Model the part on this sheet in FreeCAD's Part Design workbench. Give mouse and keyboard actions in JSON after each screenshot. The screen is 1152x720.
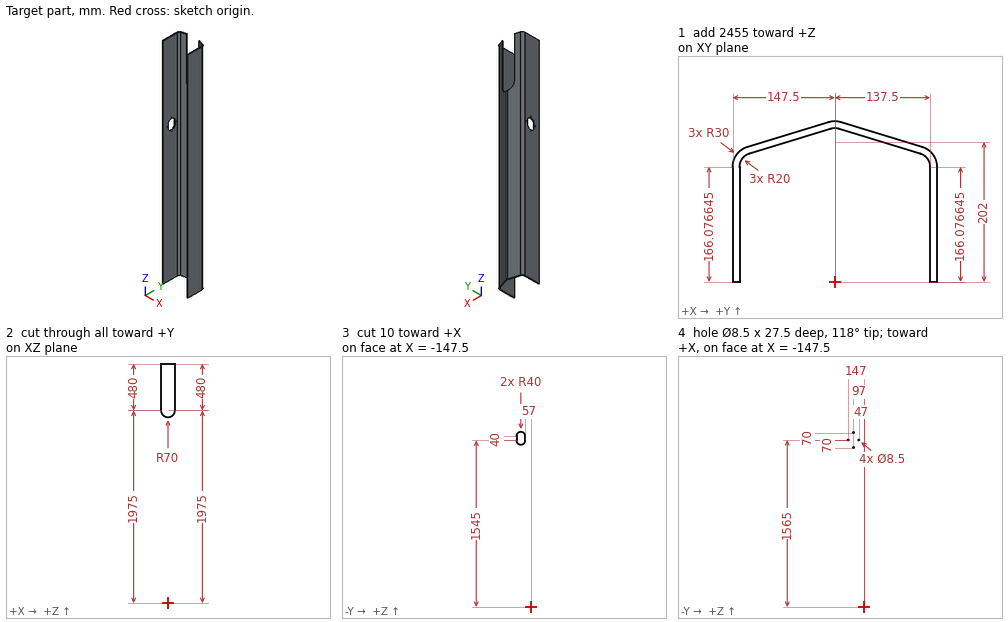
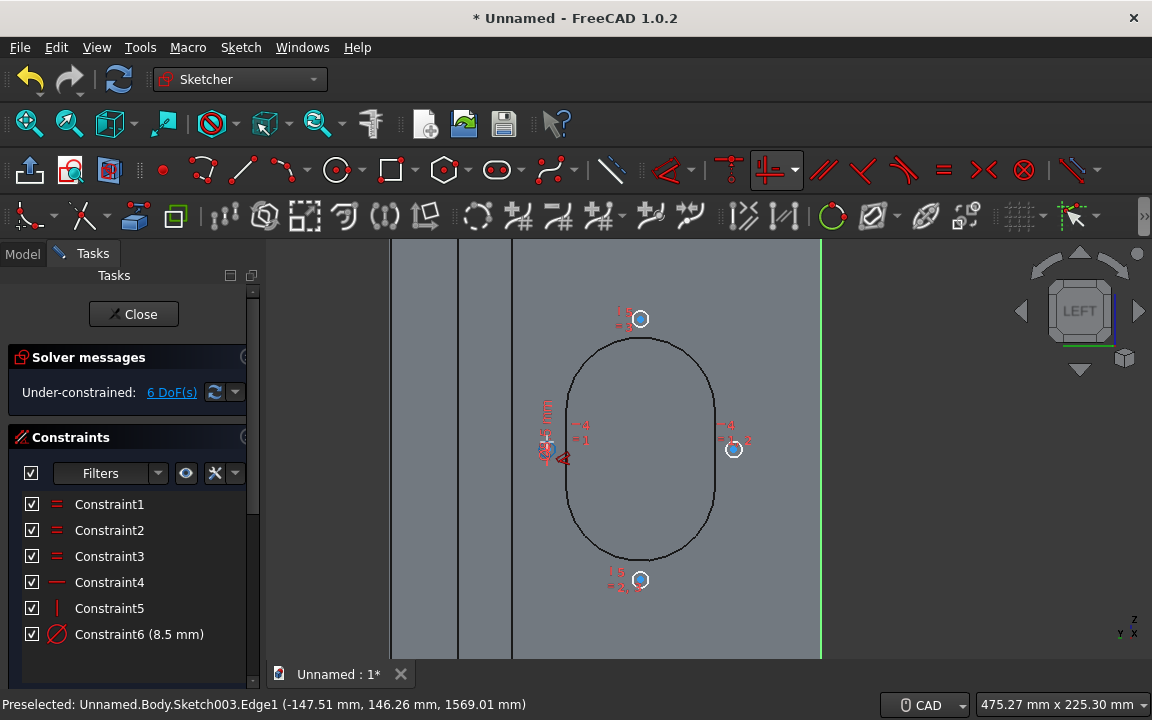
{"action": "left_click", "coordinate": [734, 449]}
{"action": "left_click", "coordinate": [778, 415]}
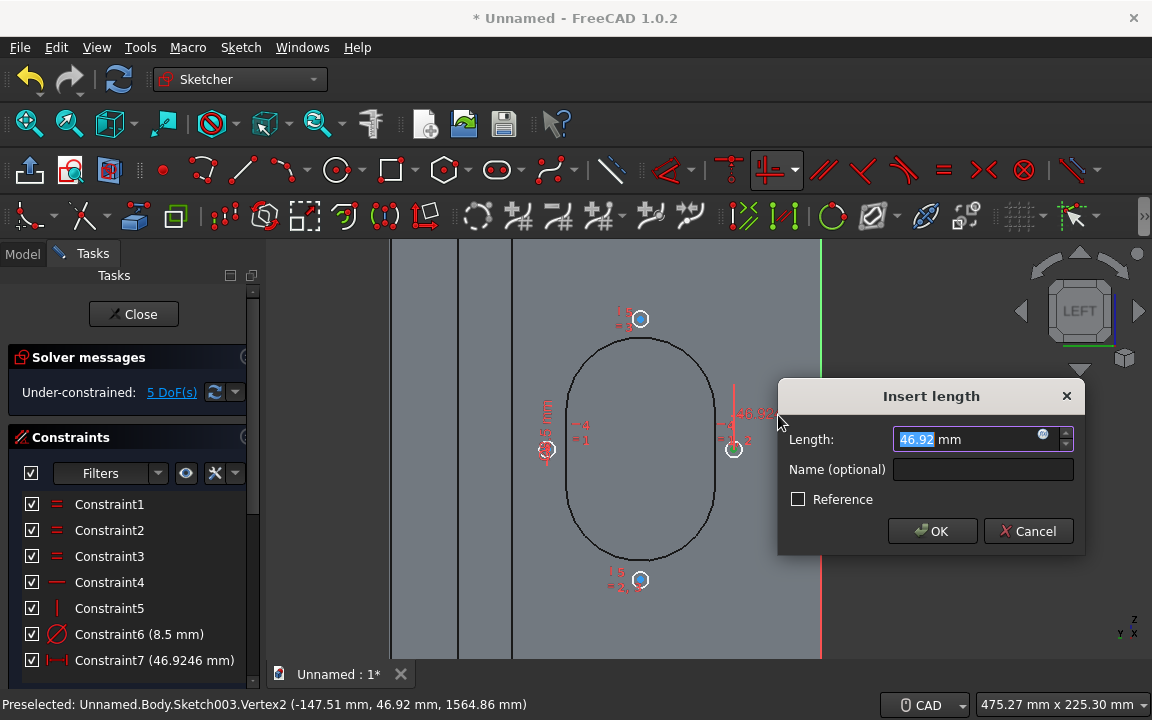
{"action": "type", "text": "47"}
{"action": "key", "text": "Return"}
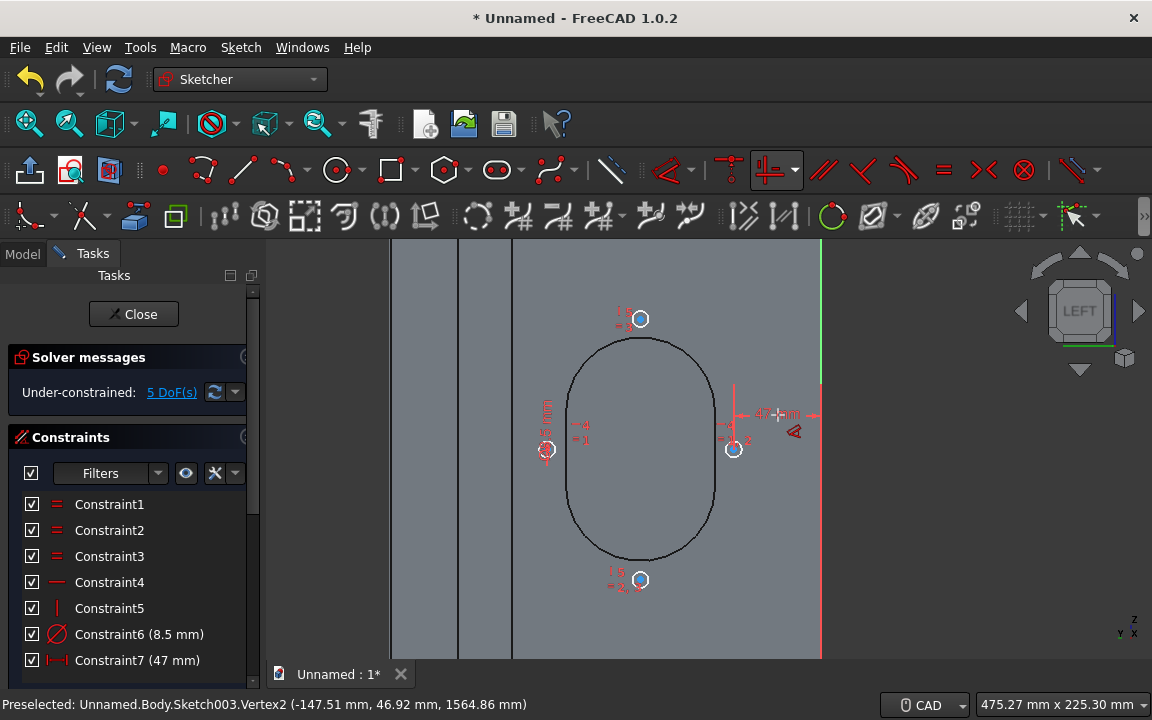
{"action": "left_click", "coordinate": [641, 580]}
{"action": "left_click", "coordinate": [731, 546]}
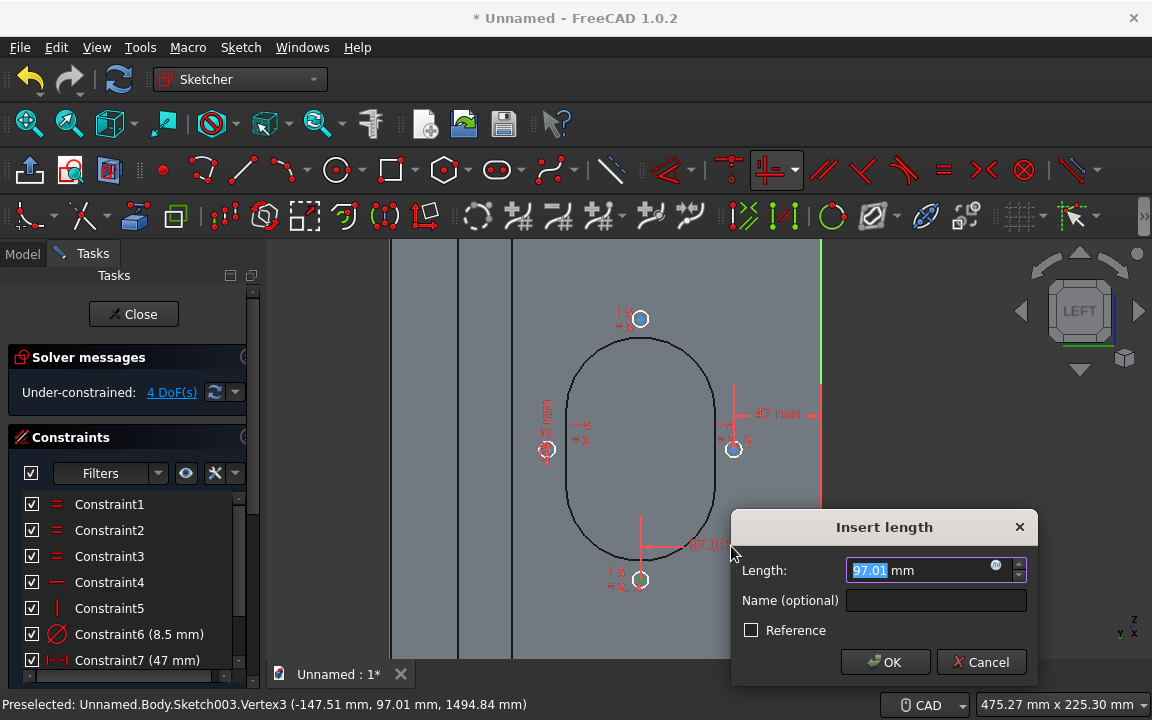
{"action": "type", "text": "97"}
{"action": "key", "text": "Return"}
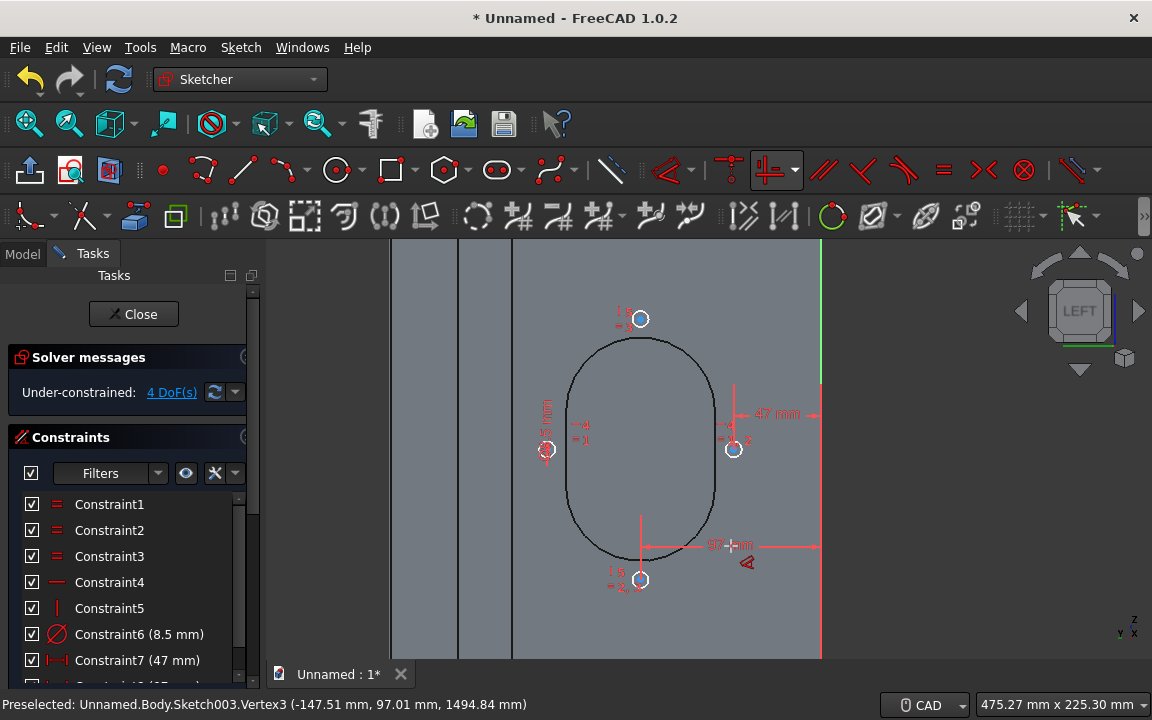
{"action": "left_click", "coordinate": [547, 449]}
{"action": "left_click", "coordinate": [684, 415]}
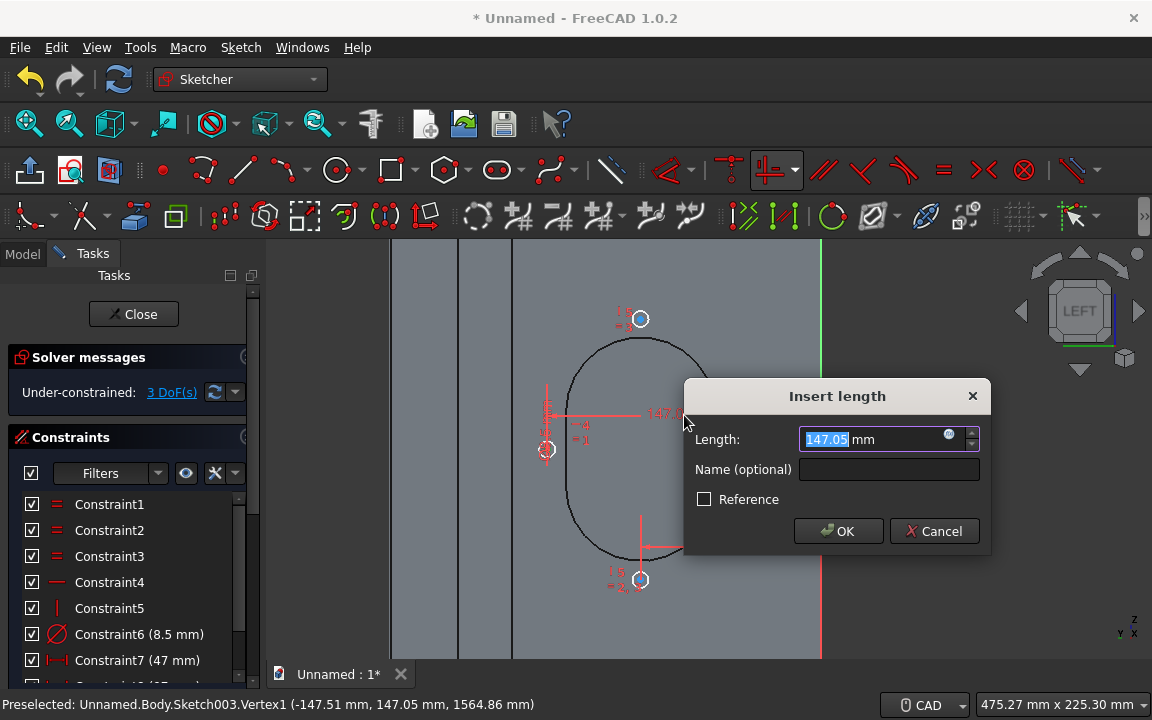
{"action": "type", "text": "147"}
{"action": "key", "text": "Return"}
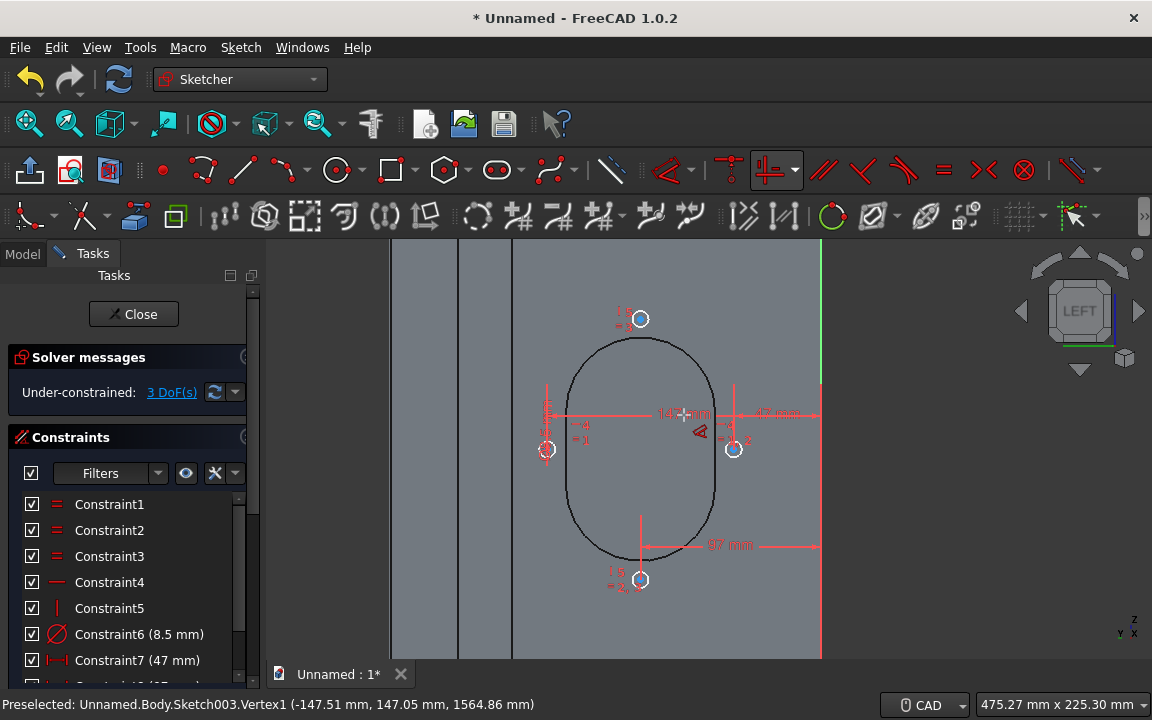
{"action": "left_click", "coordinate": [547, 449]}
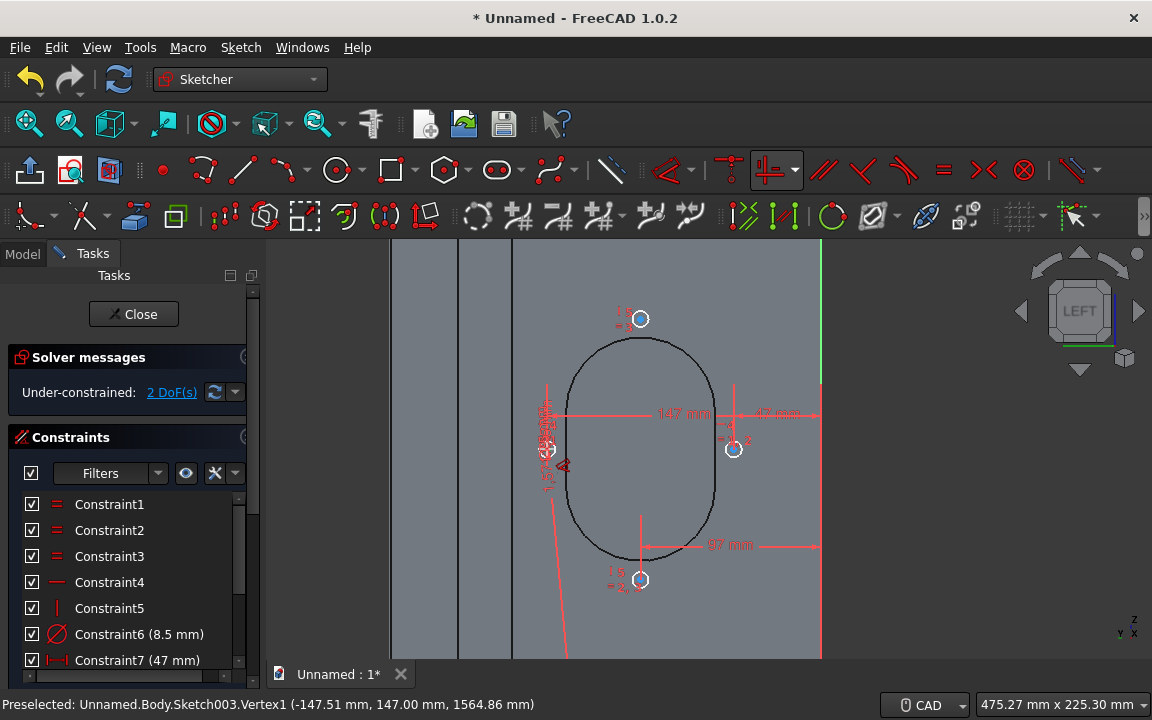
{"action": "left_click", "coordinate": [641, 580]}
{"action": "left_click", "coordinate": [513, 515]}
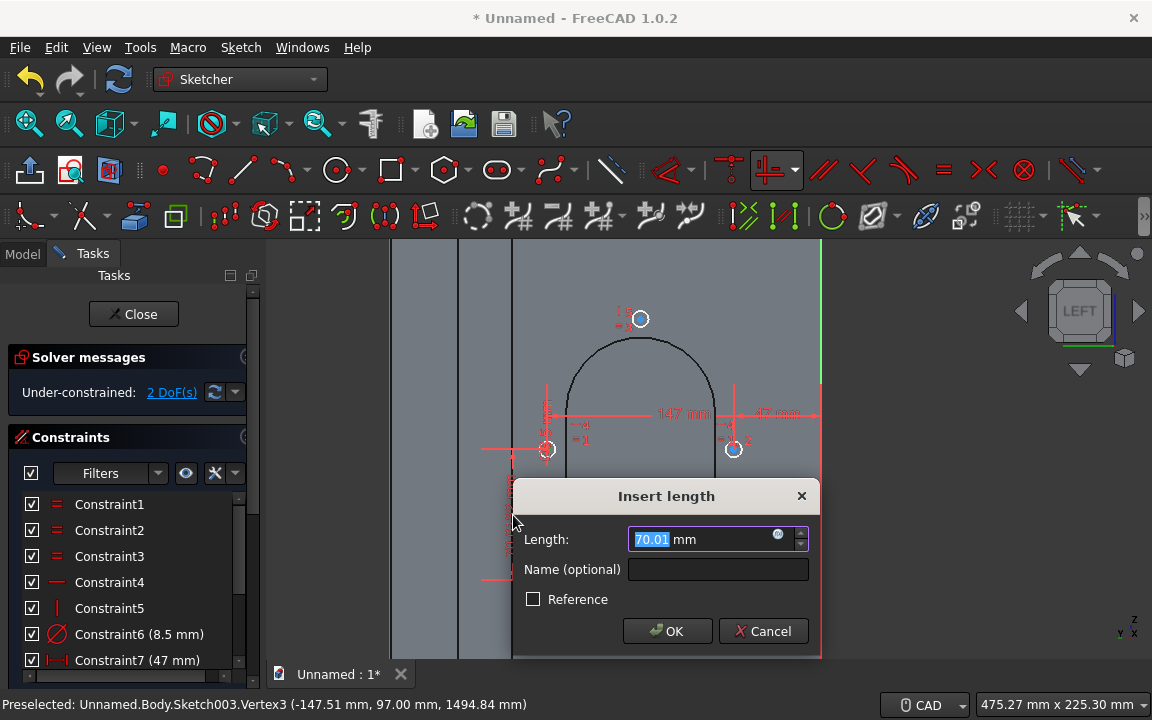
{"action": "type", "text": "70"}
{"action": "key", "text": "Return"}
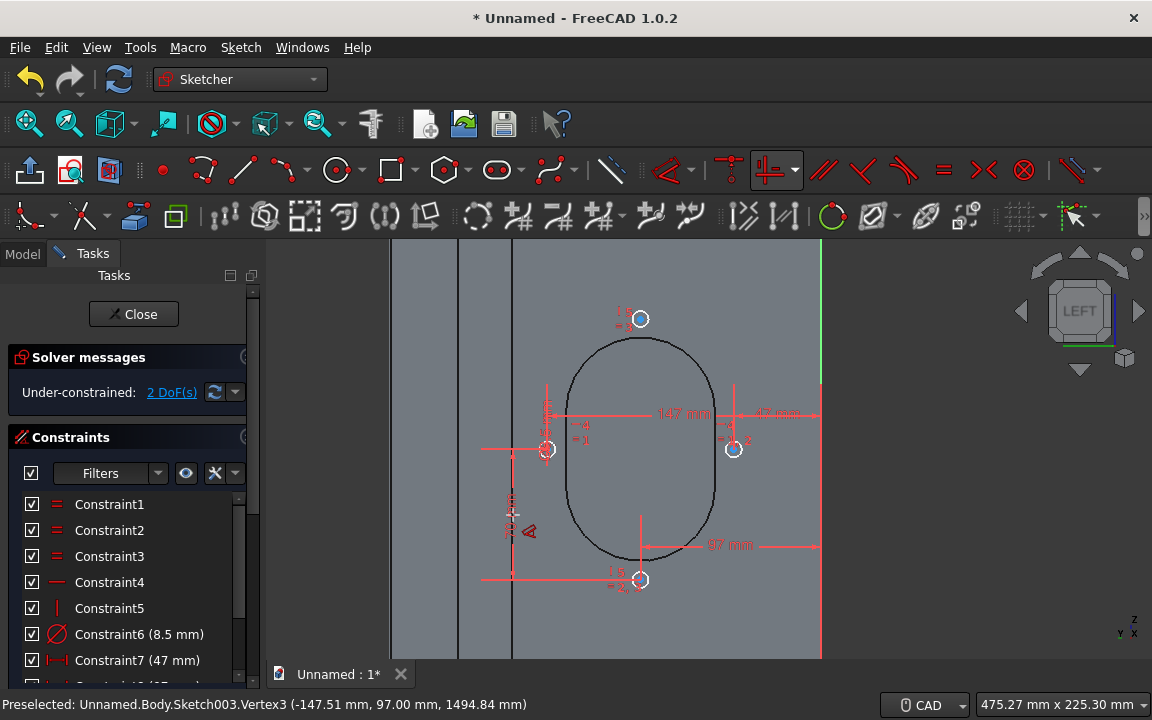
{"action": "left_click", "coordinate": [547, 449]}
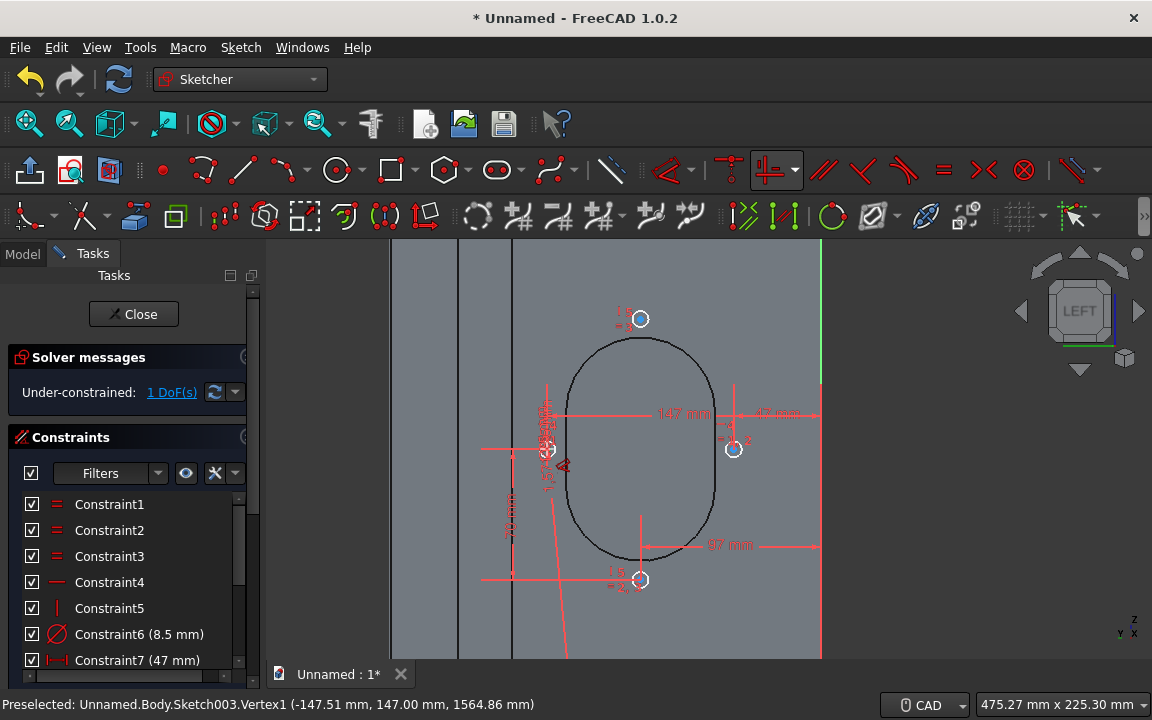
{"action": "left_click", "coordinate": [641, 319]}
{"action": "left_click", "coordinate": [513, 384]}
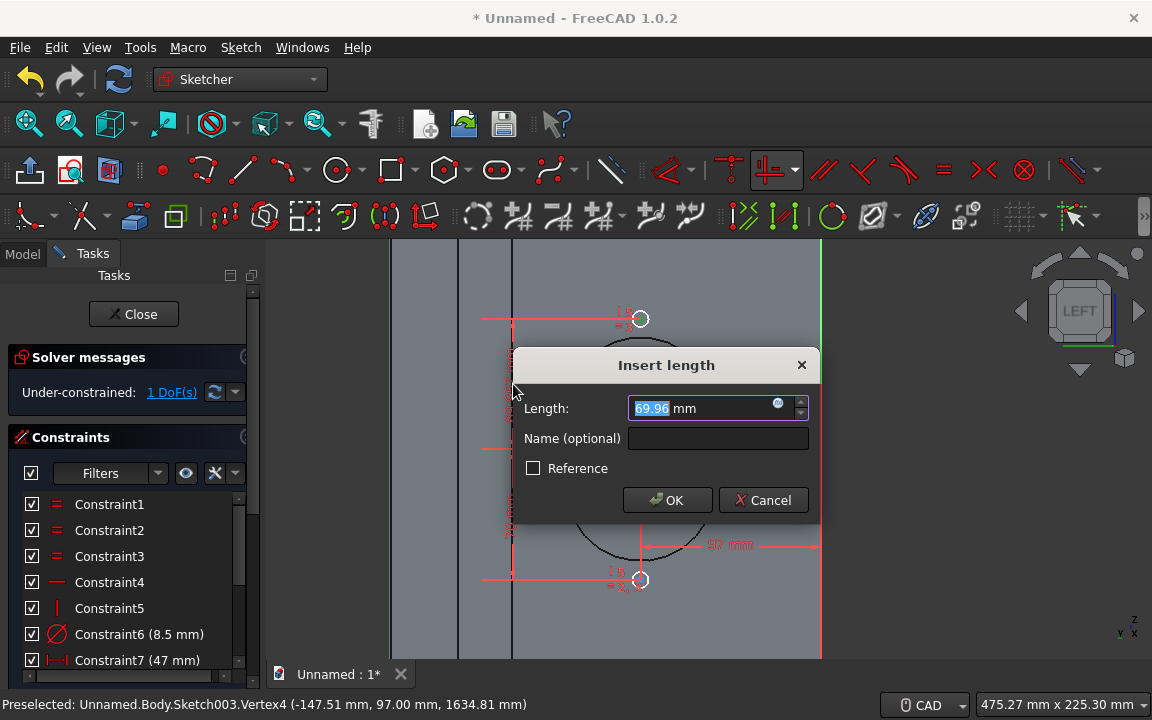
{"action": "type", "text": "70"}
{"action": "key", "text": "Return"}